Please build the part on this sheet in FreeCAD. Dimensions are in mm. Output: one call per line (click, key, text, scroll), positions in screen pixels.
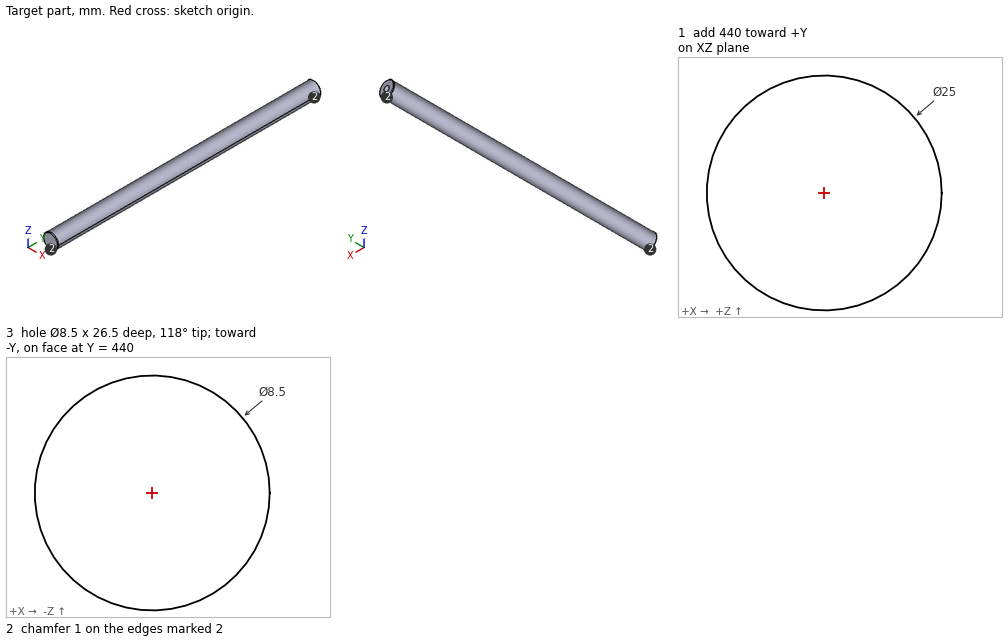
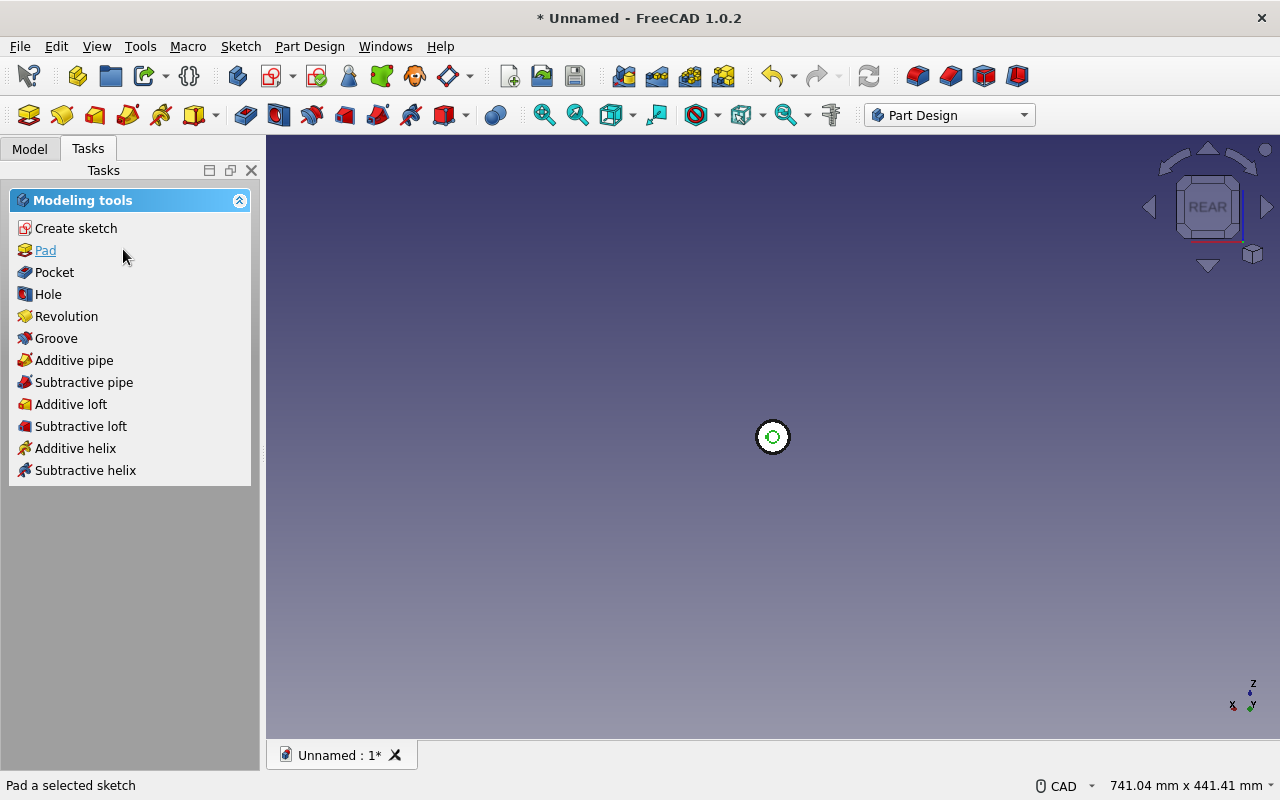
click(279, 116)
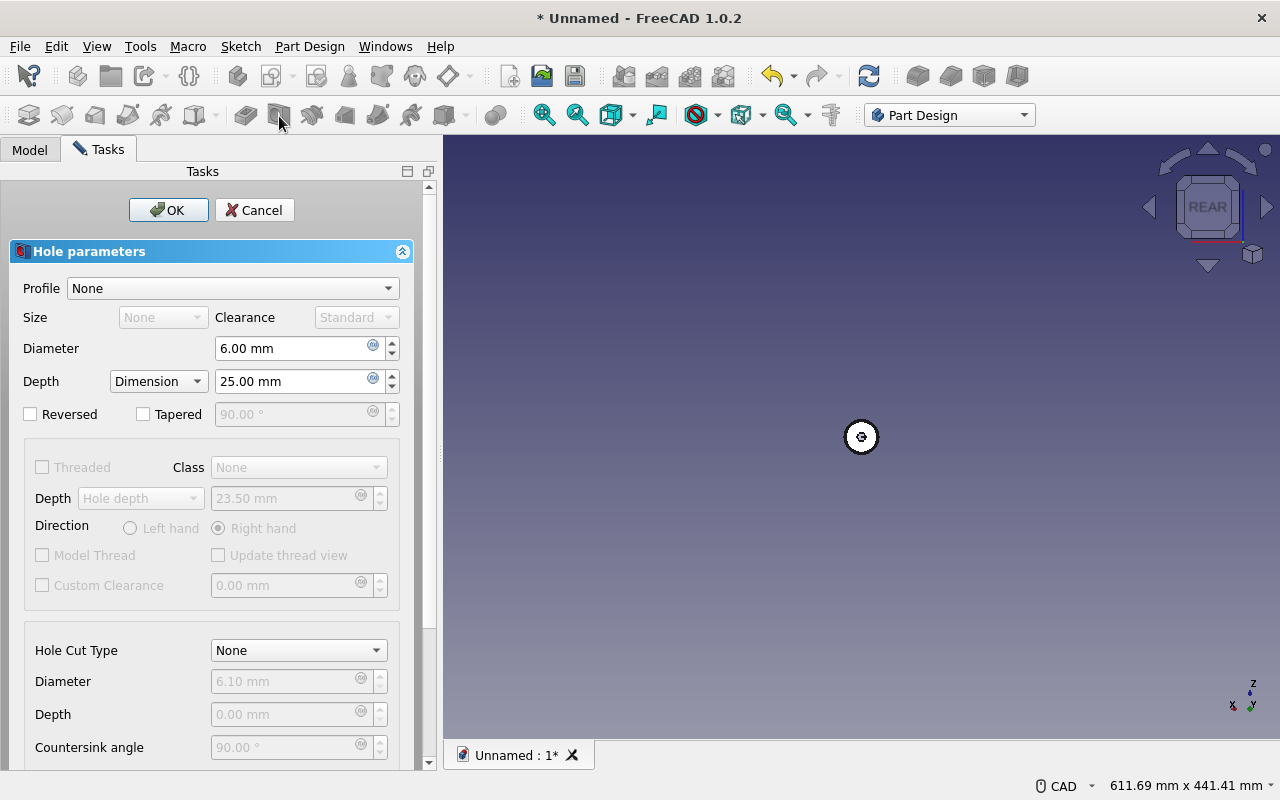
triple_click(300, 348)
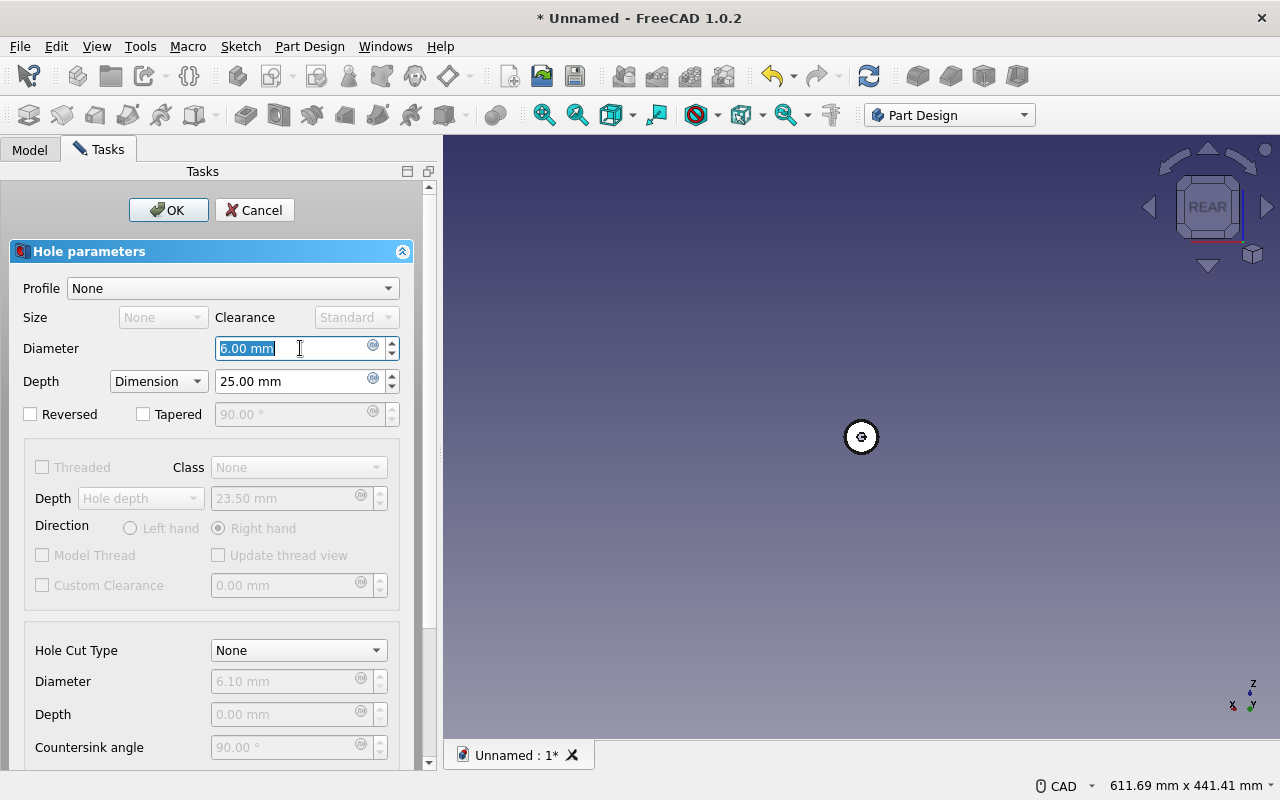
text(8.5)
key(Tab)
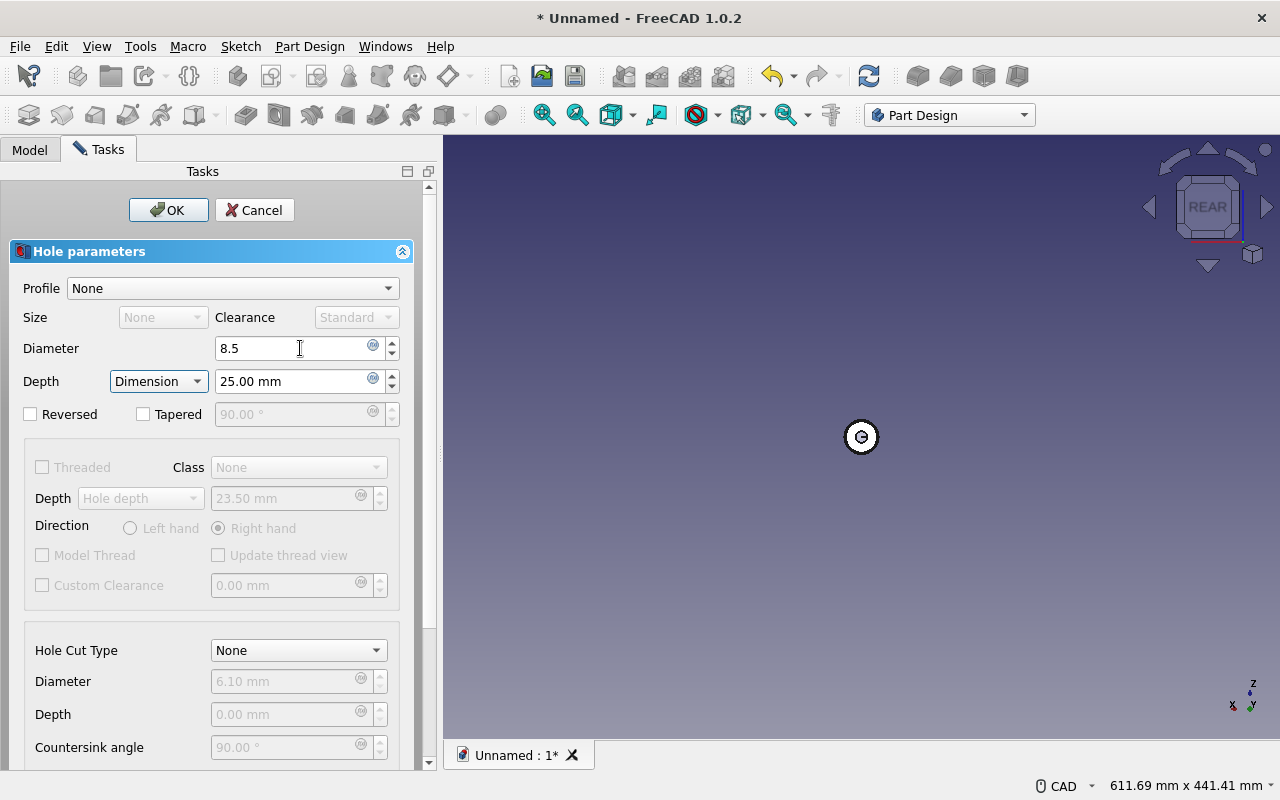
triple_click(300, 382)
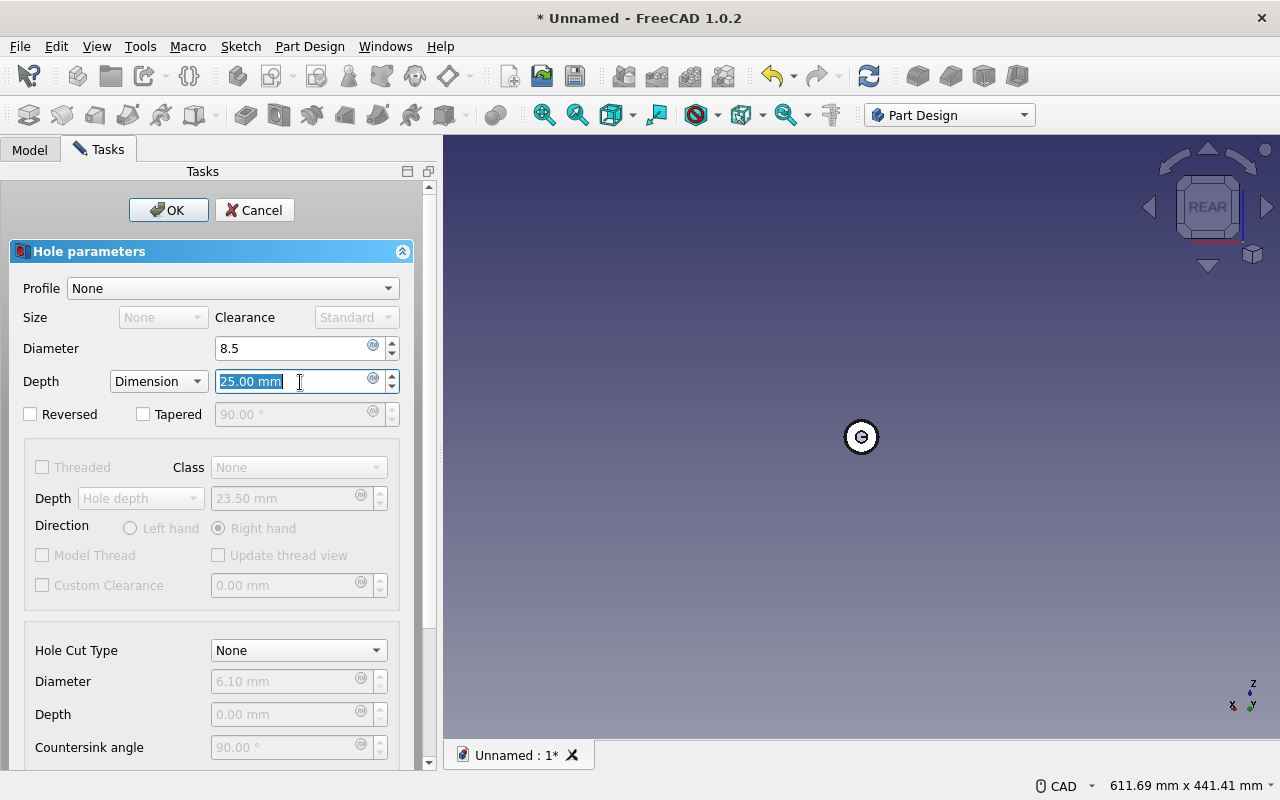
text(26.5)
key(Tab)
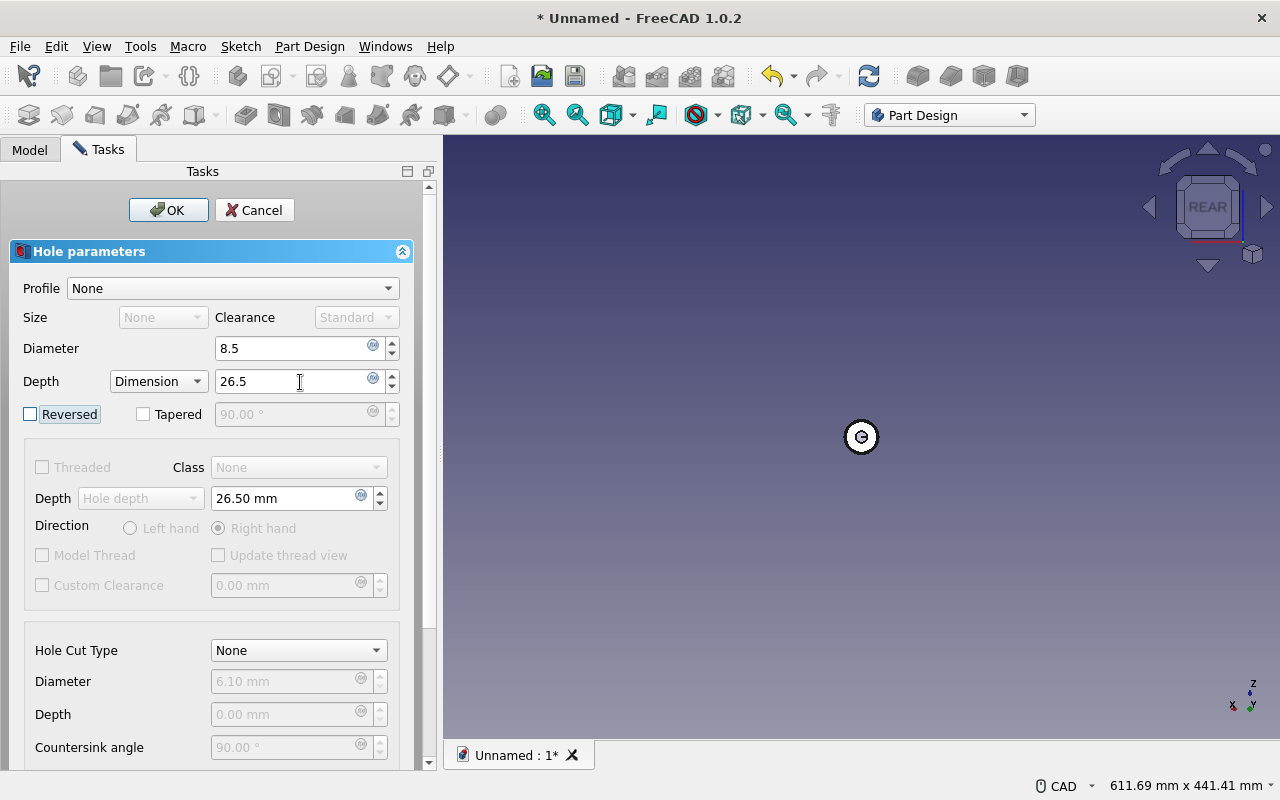
click(169, 210)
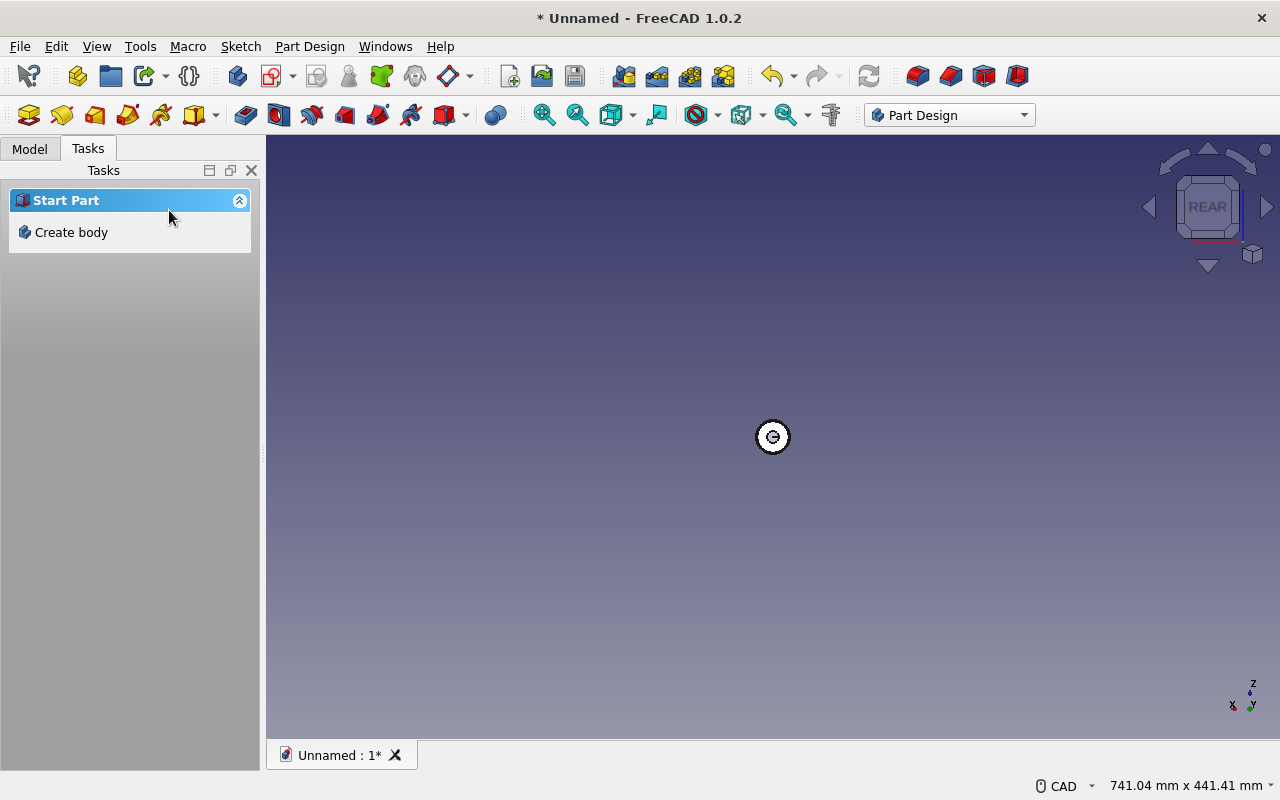
key(0)